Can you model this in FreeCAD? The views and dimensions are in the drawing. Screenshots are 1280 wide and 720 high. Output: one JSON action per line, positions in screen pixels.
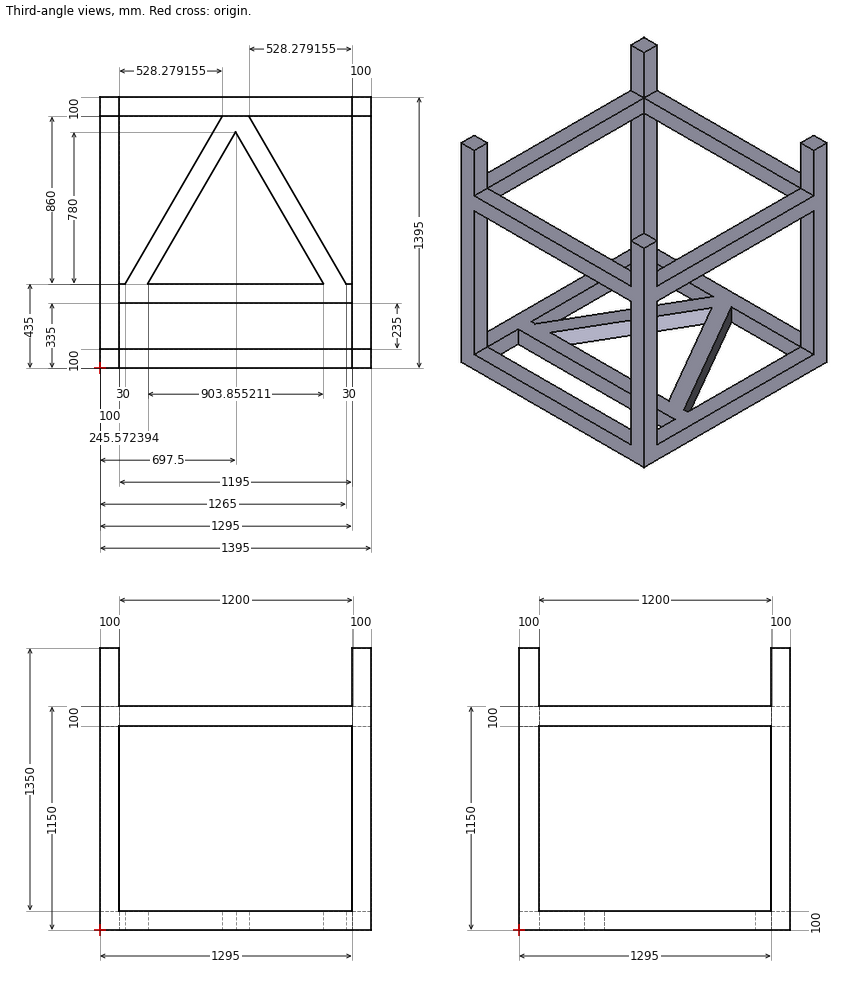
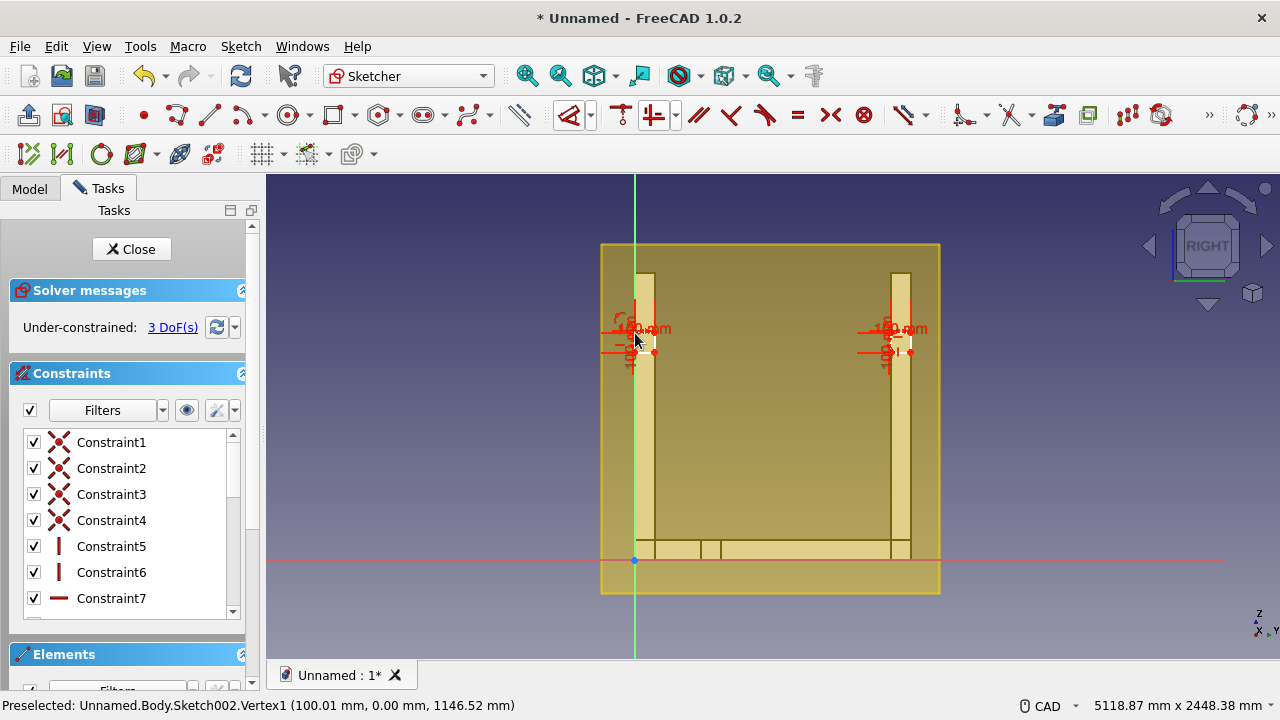
{"action": "left_click", "coordinate": [590, 116]}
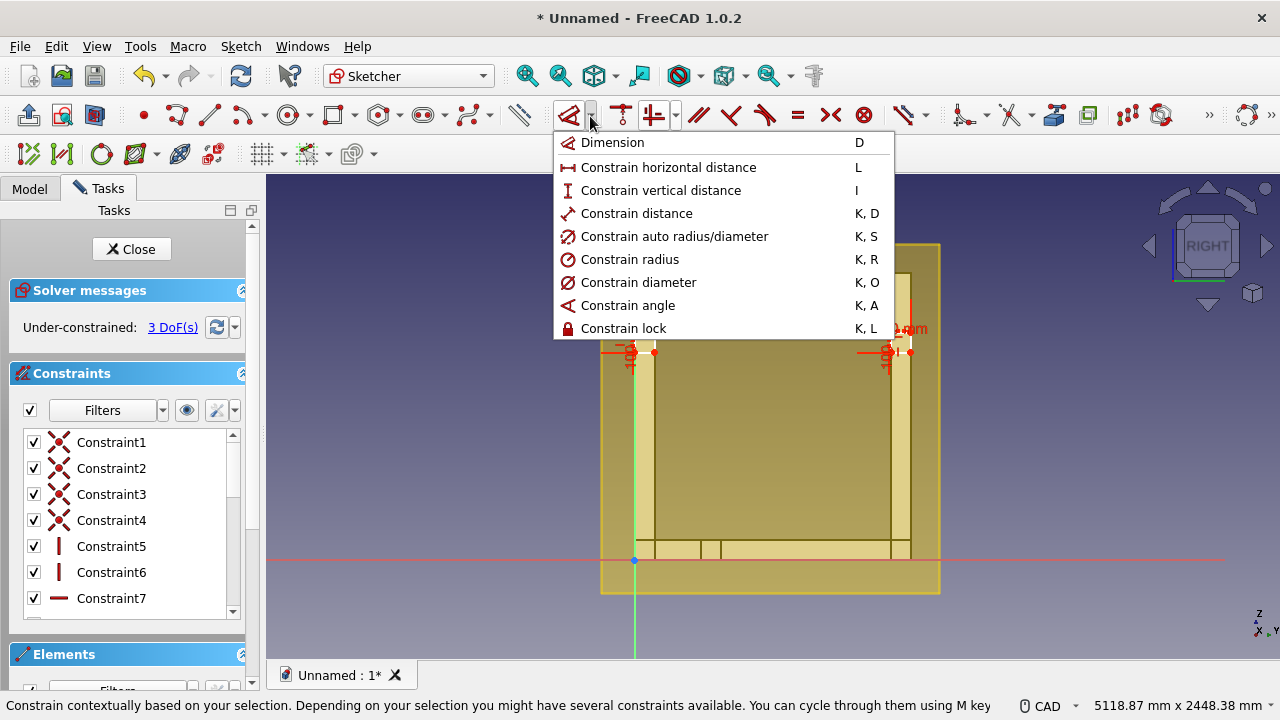
{"action": "left_click", "coordinate": [724, 190]}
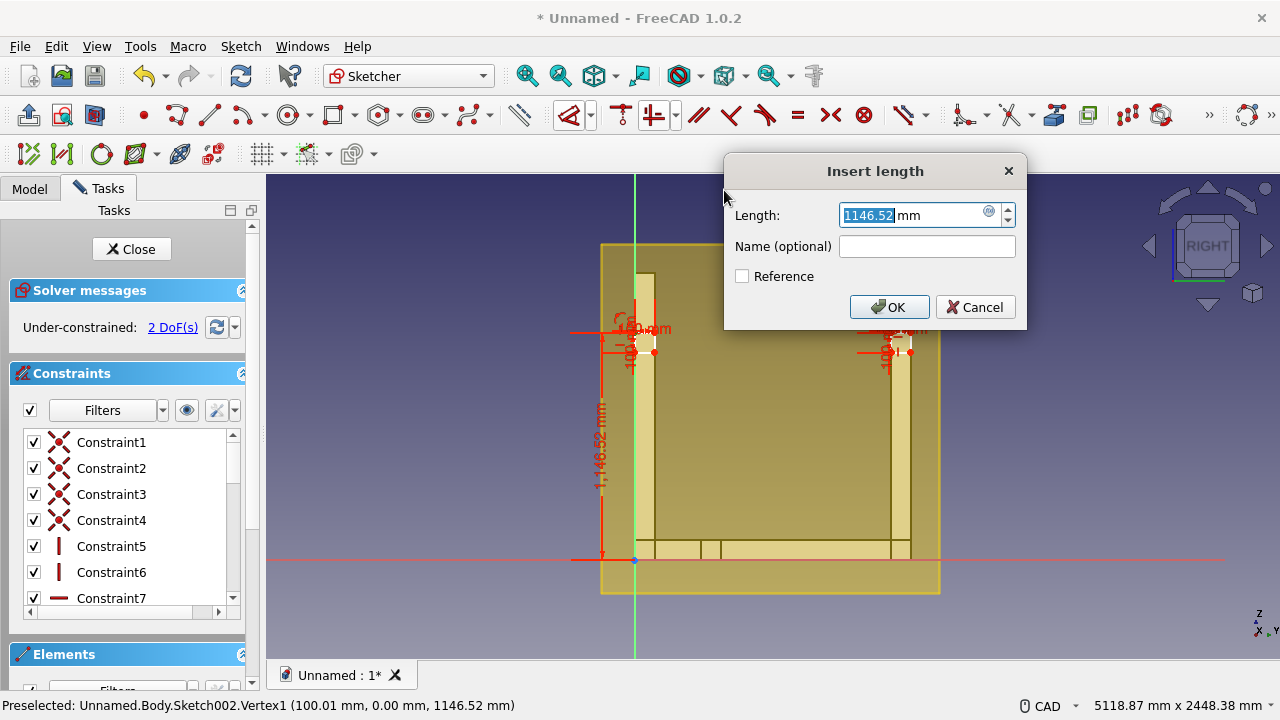
{"action": "type", "text": "1150"}
{"action": "key", "text": "Return"}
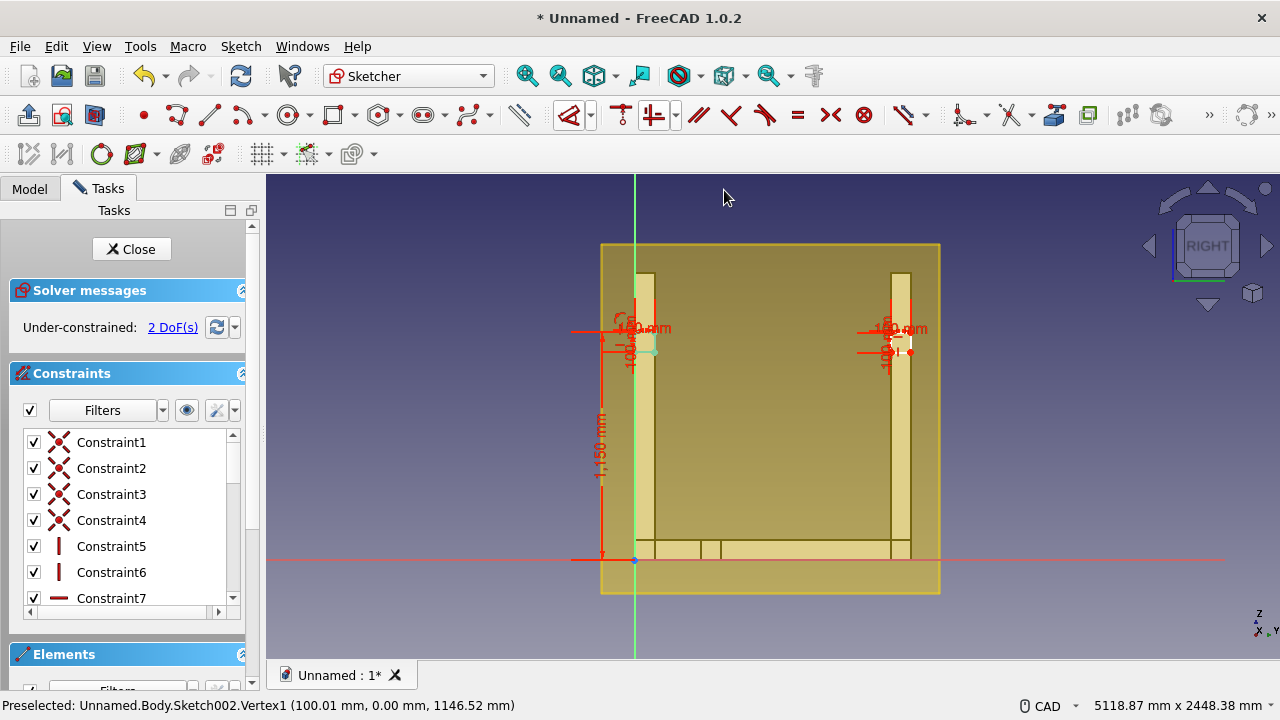
{"action": "left_click", "coordinate": [891, 333]}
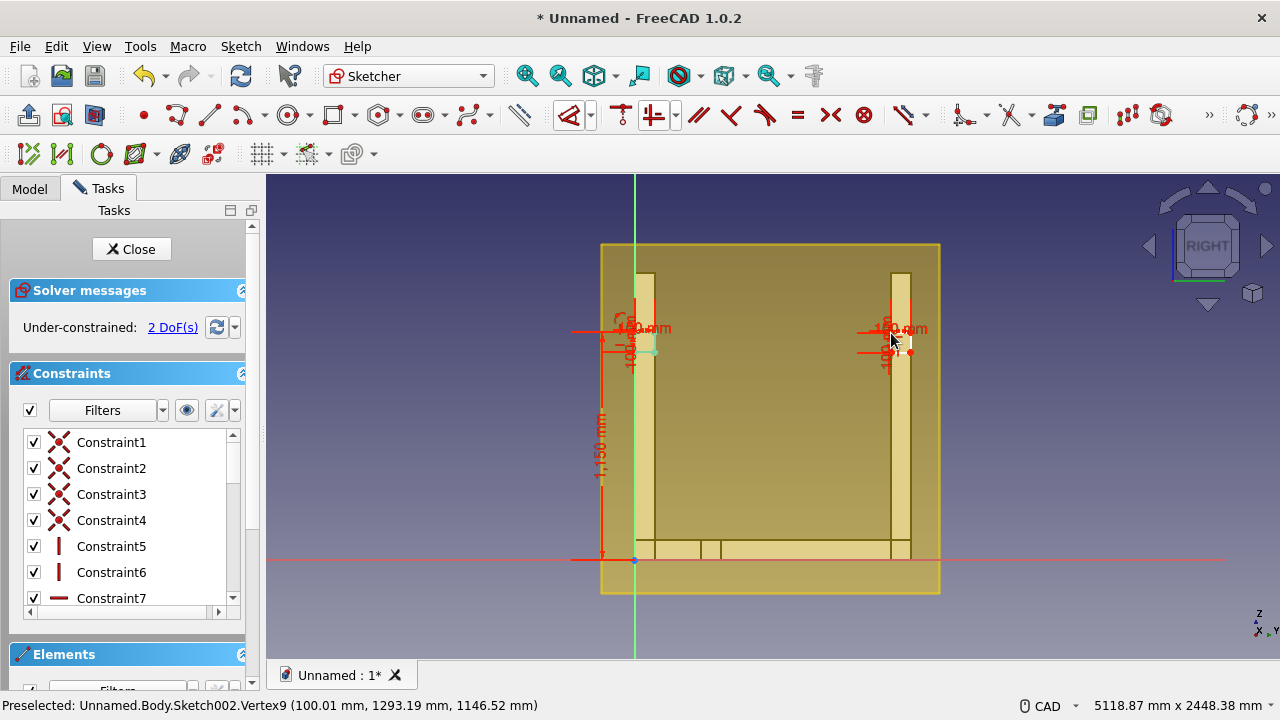
{"action": "key", "text": "l"}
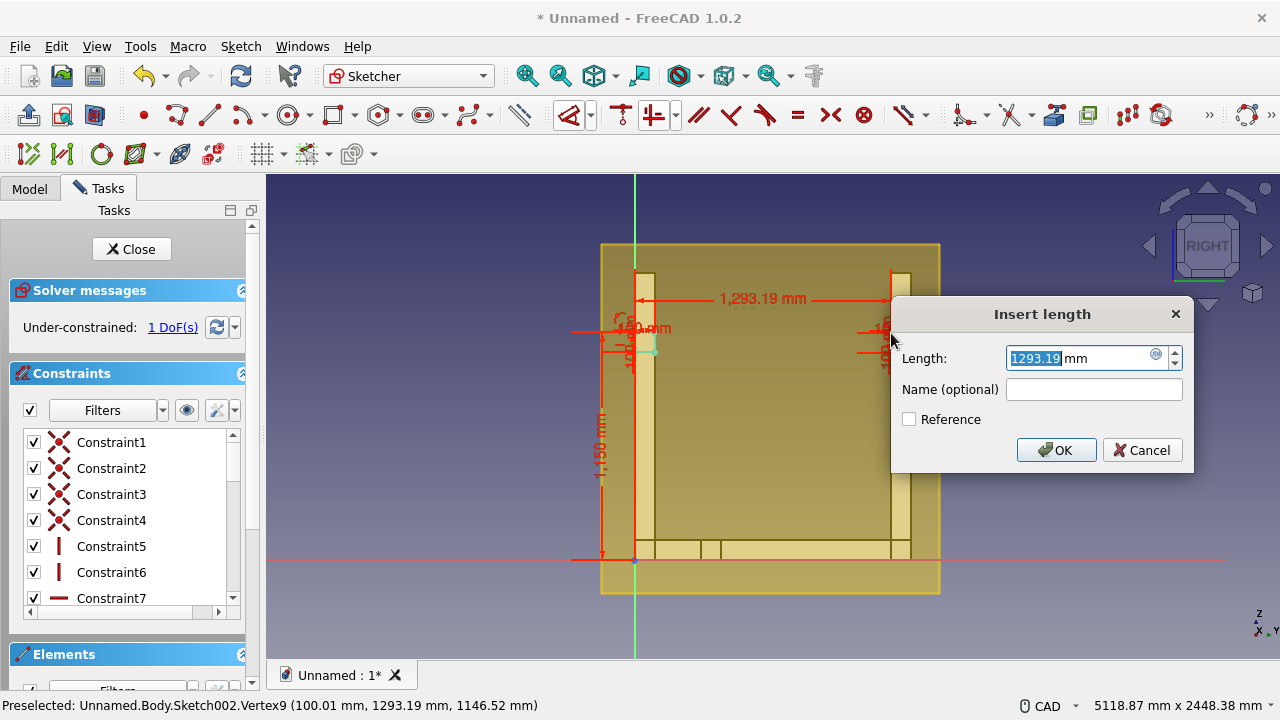
{"action": "type", "text": "1295"}
{"action": "key", "text": "Return"}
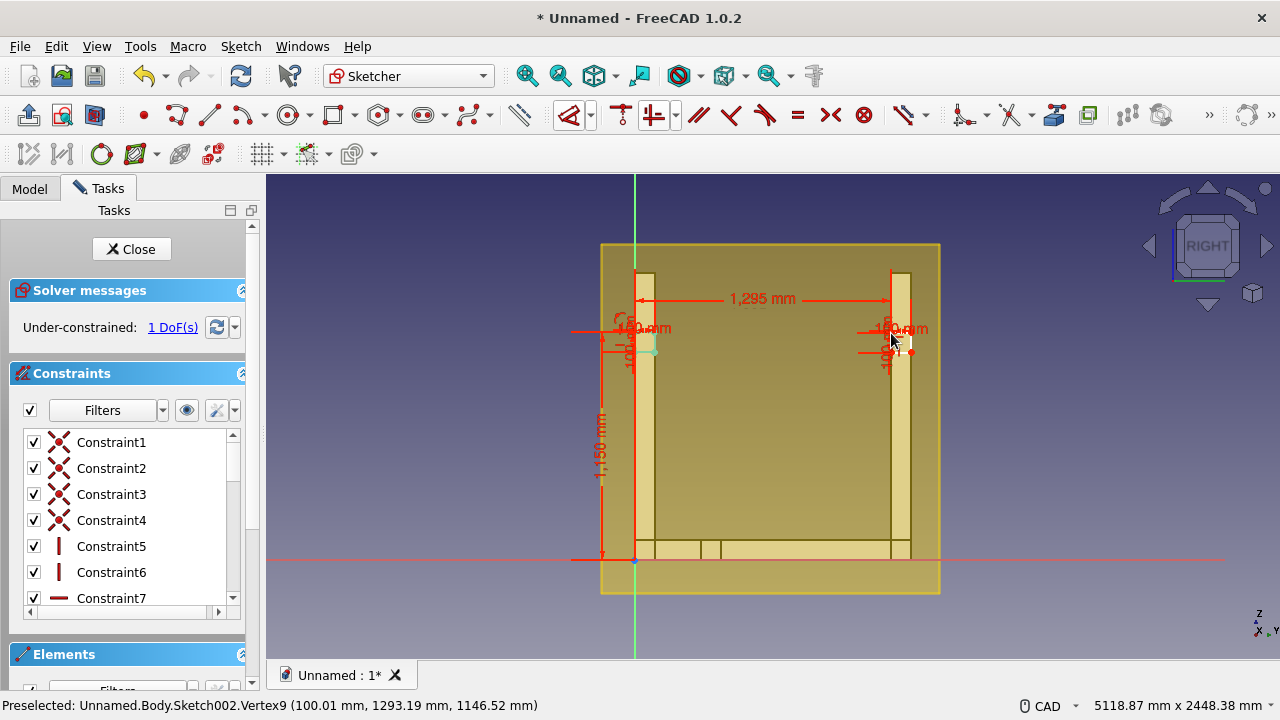
{"action": "left_click", "coordinate": [891, 333]}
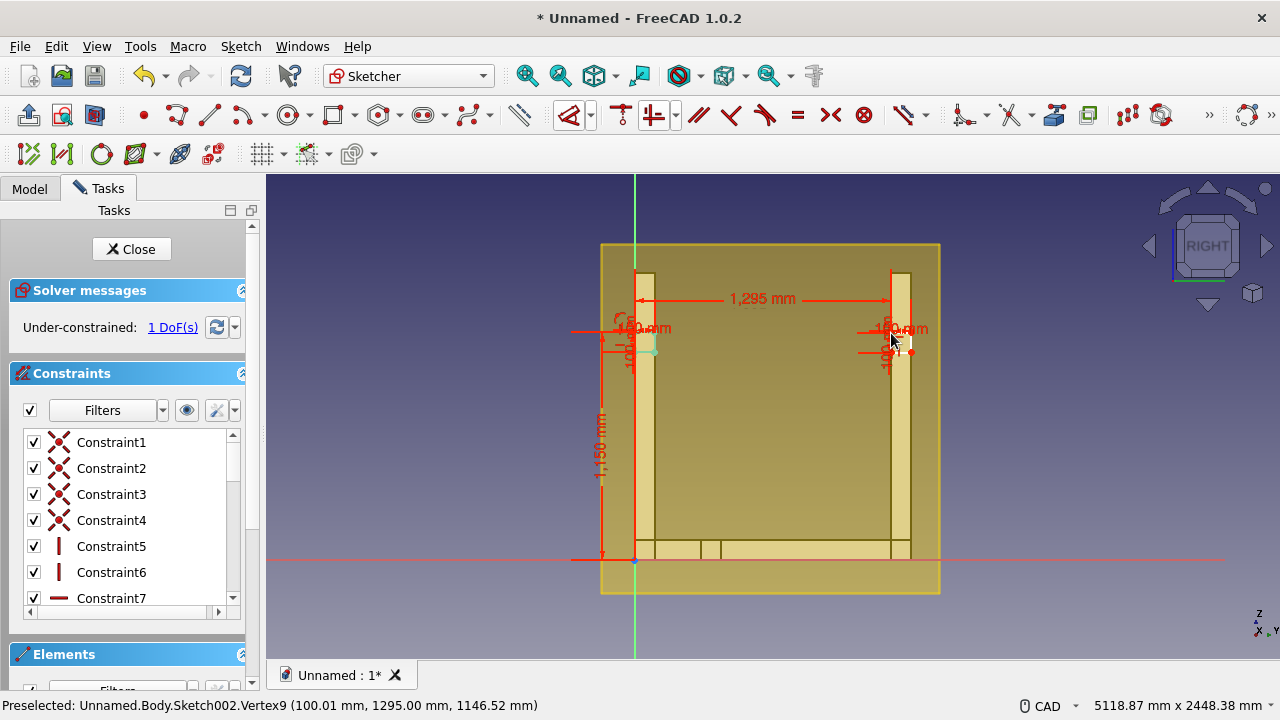
{"action": "left_click", "coordinate": [590, 116]}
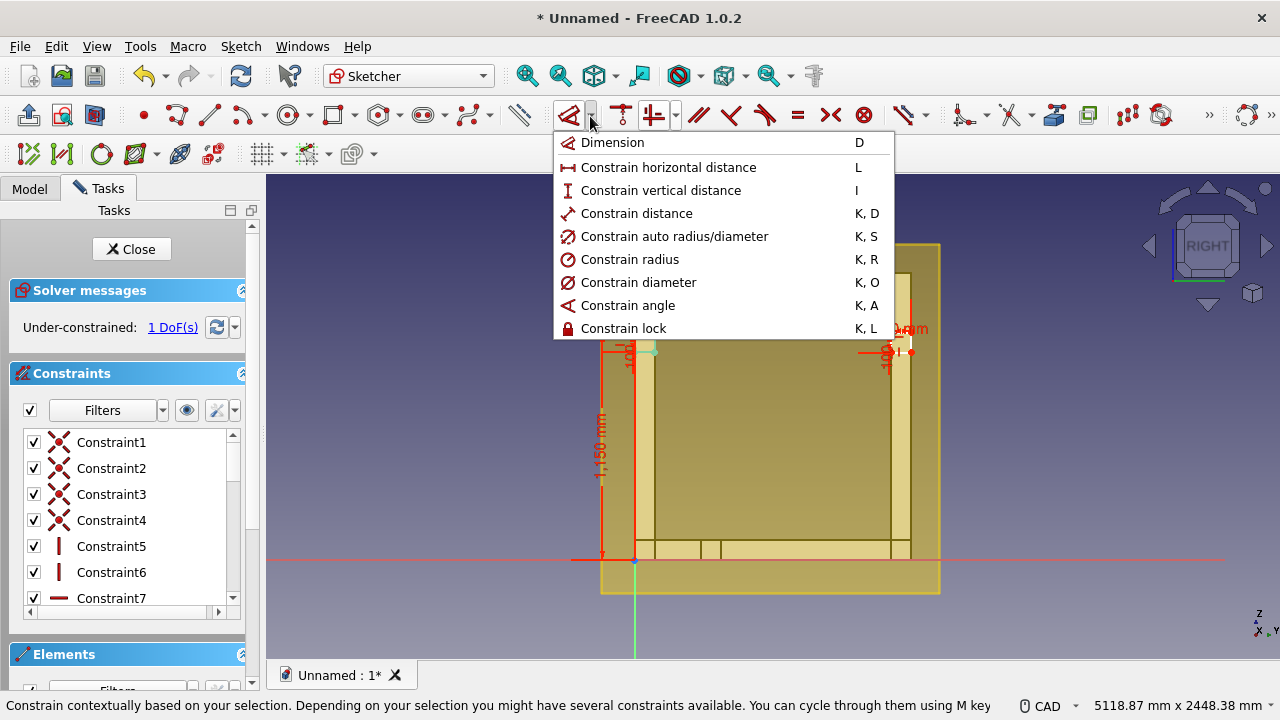
{"action": "left_click", "coordinate": [724, 190]}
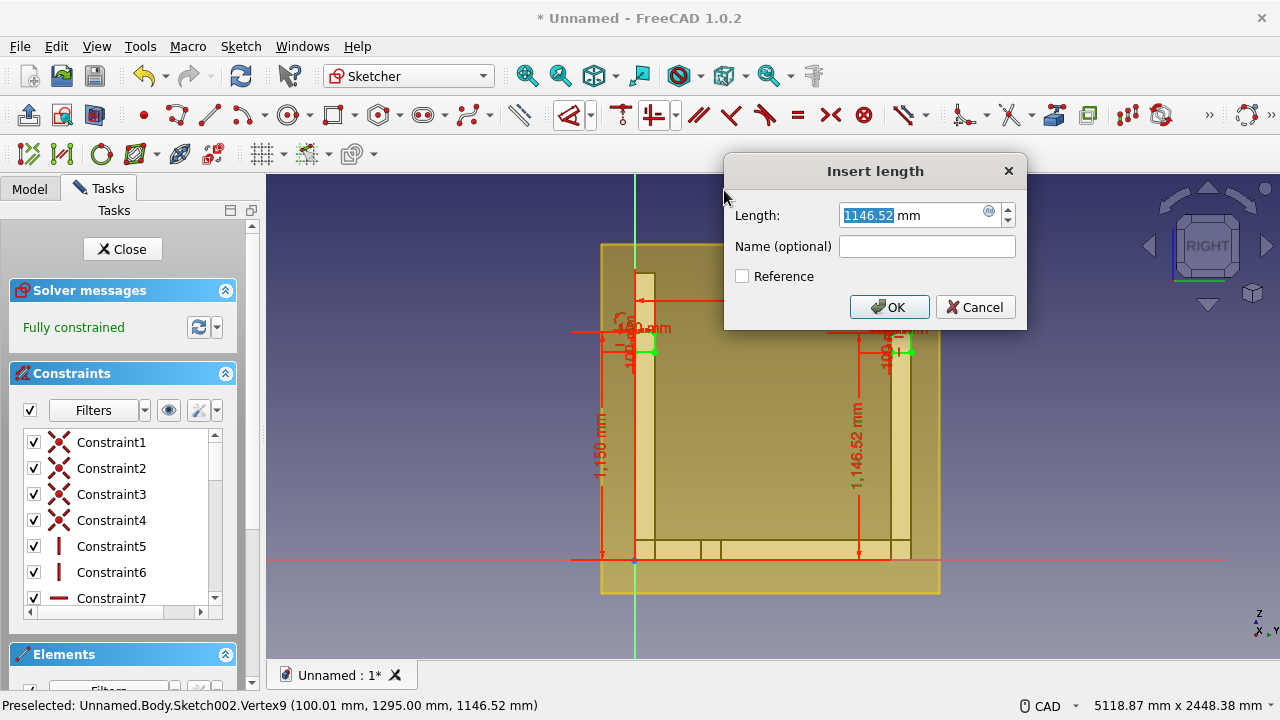
{"action": "type", "text": "1150"}
{"action": "key", "text": "Return"}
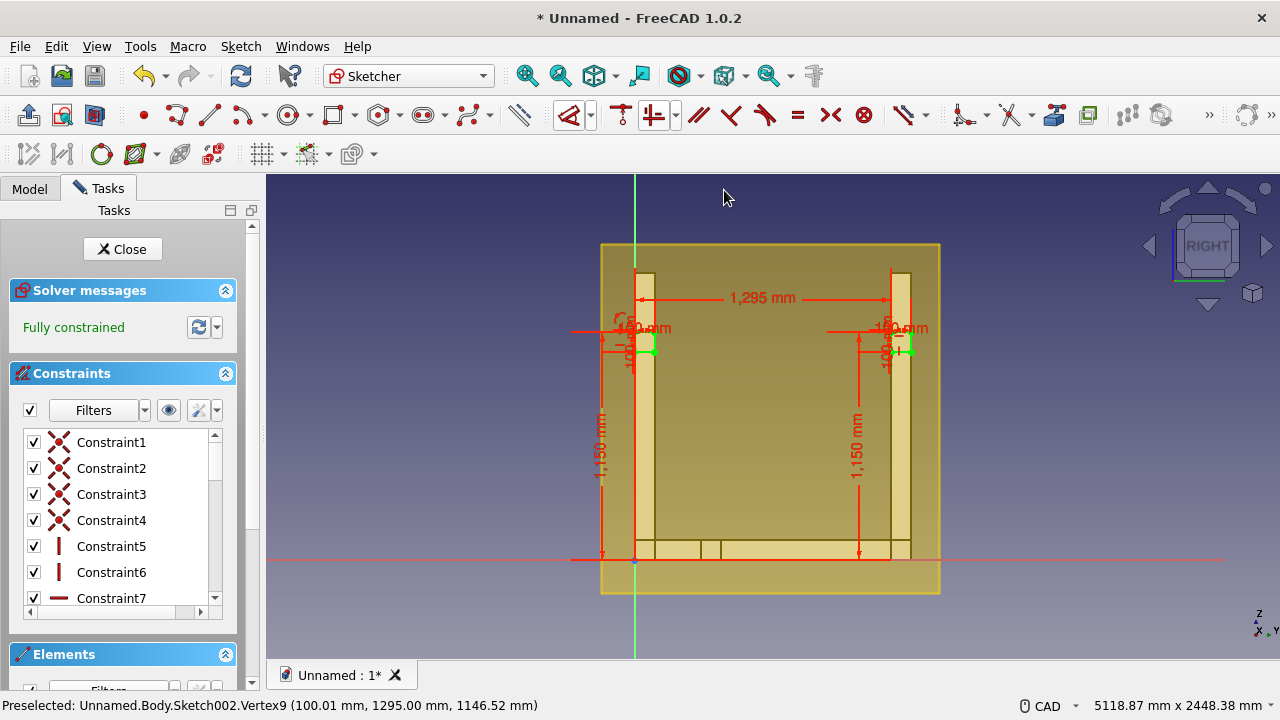
{"action": "left_click", "coordinate": [123, 249]}